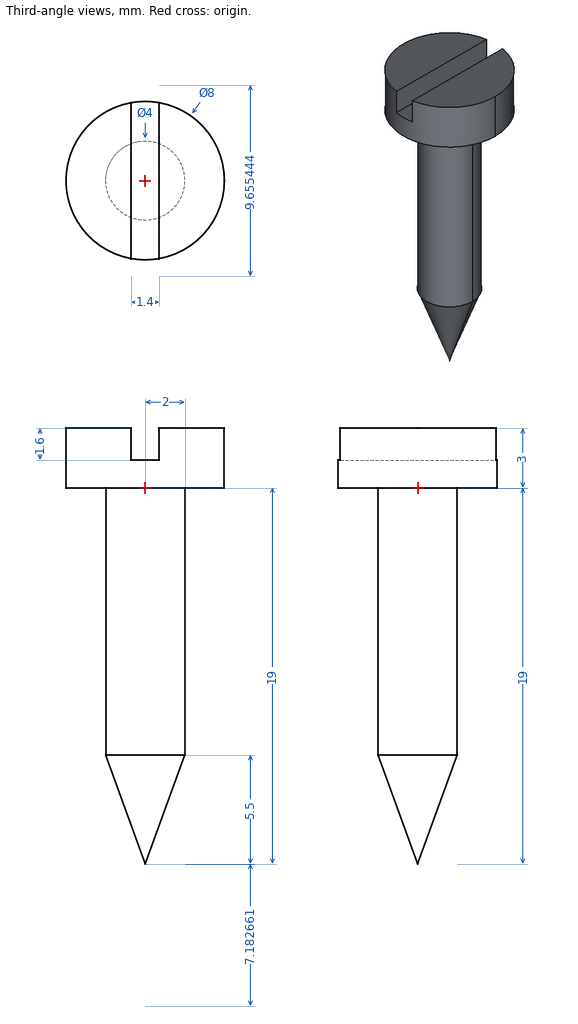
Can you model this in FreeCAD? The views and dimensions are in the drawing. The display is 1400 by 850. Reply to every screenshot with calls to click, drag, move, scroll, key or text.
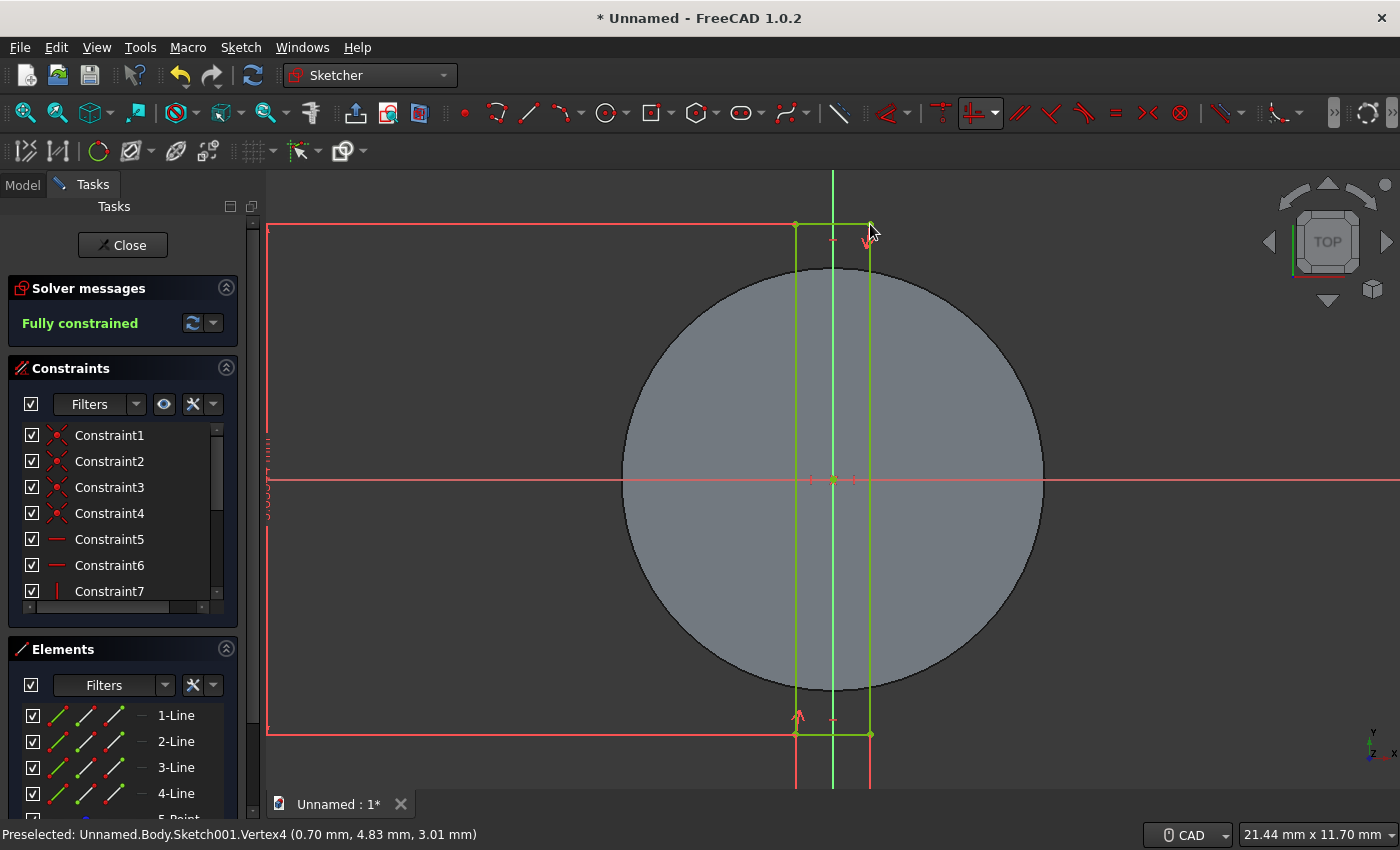
click(123, 245)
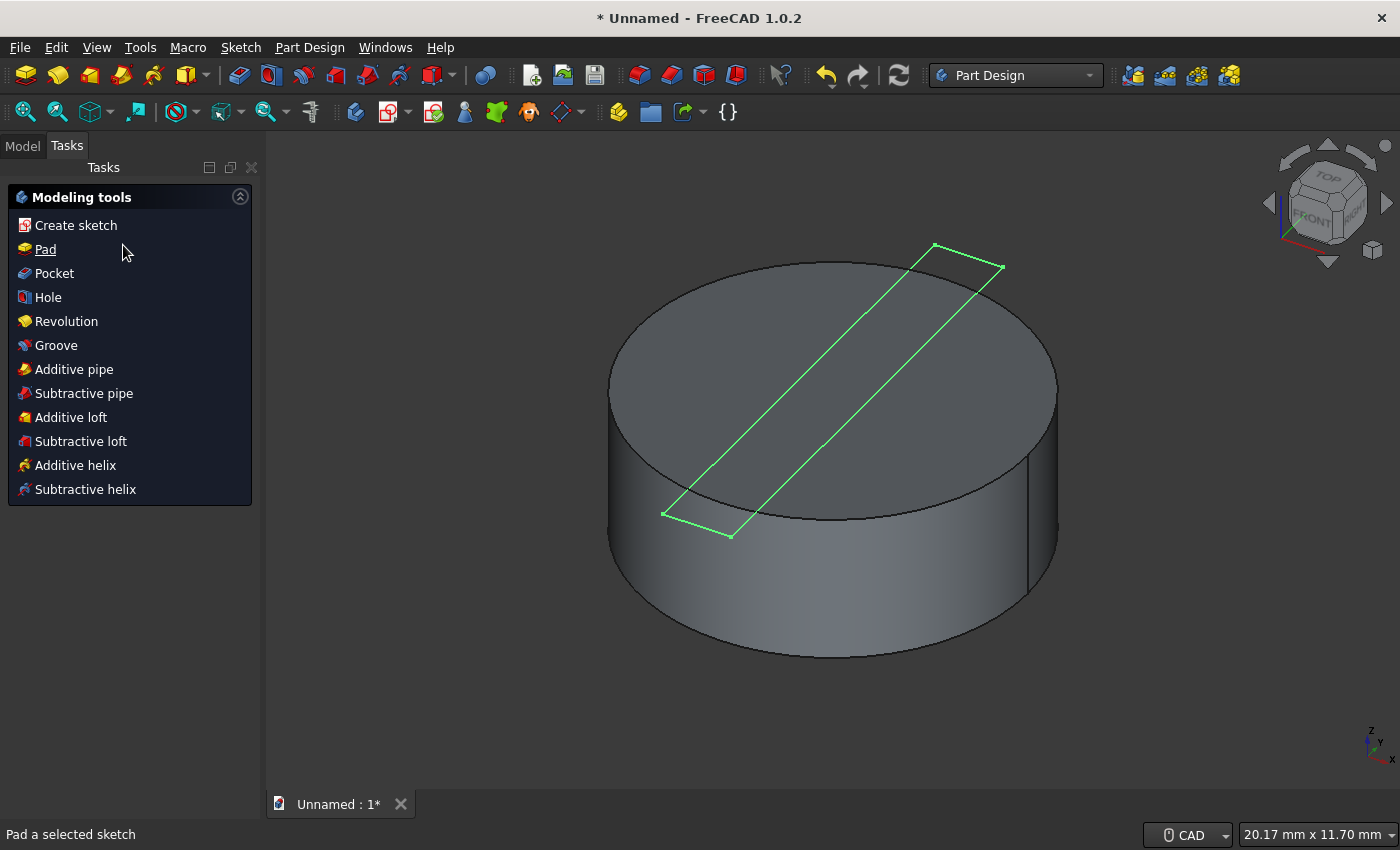
click(240, 76)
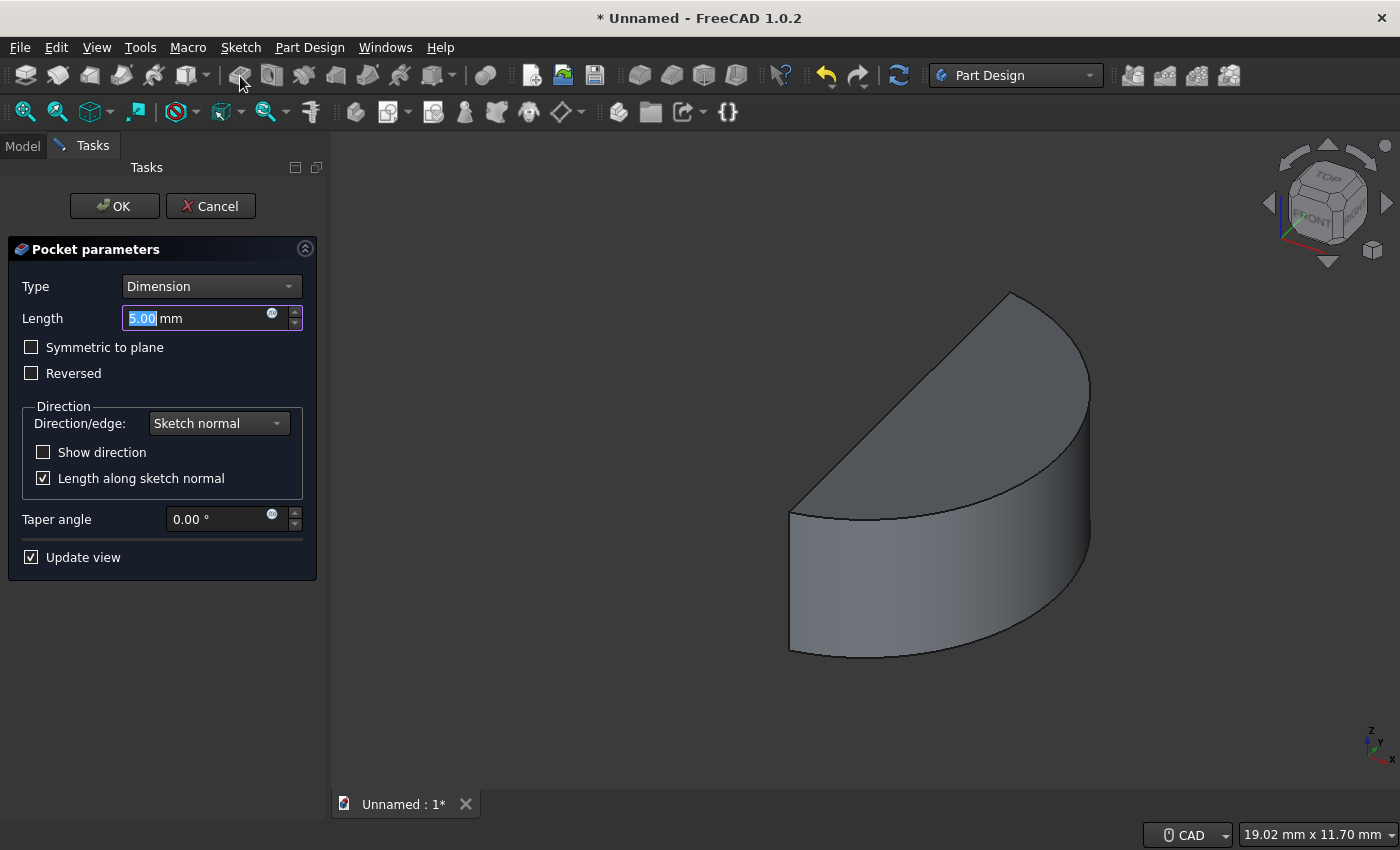
text(1.6)
key(Tab)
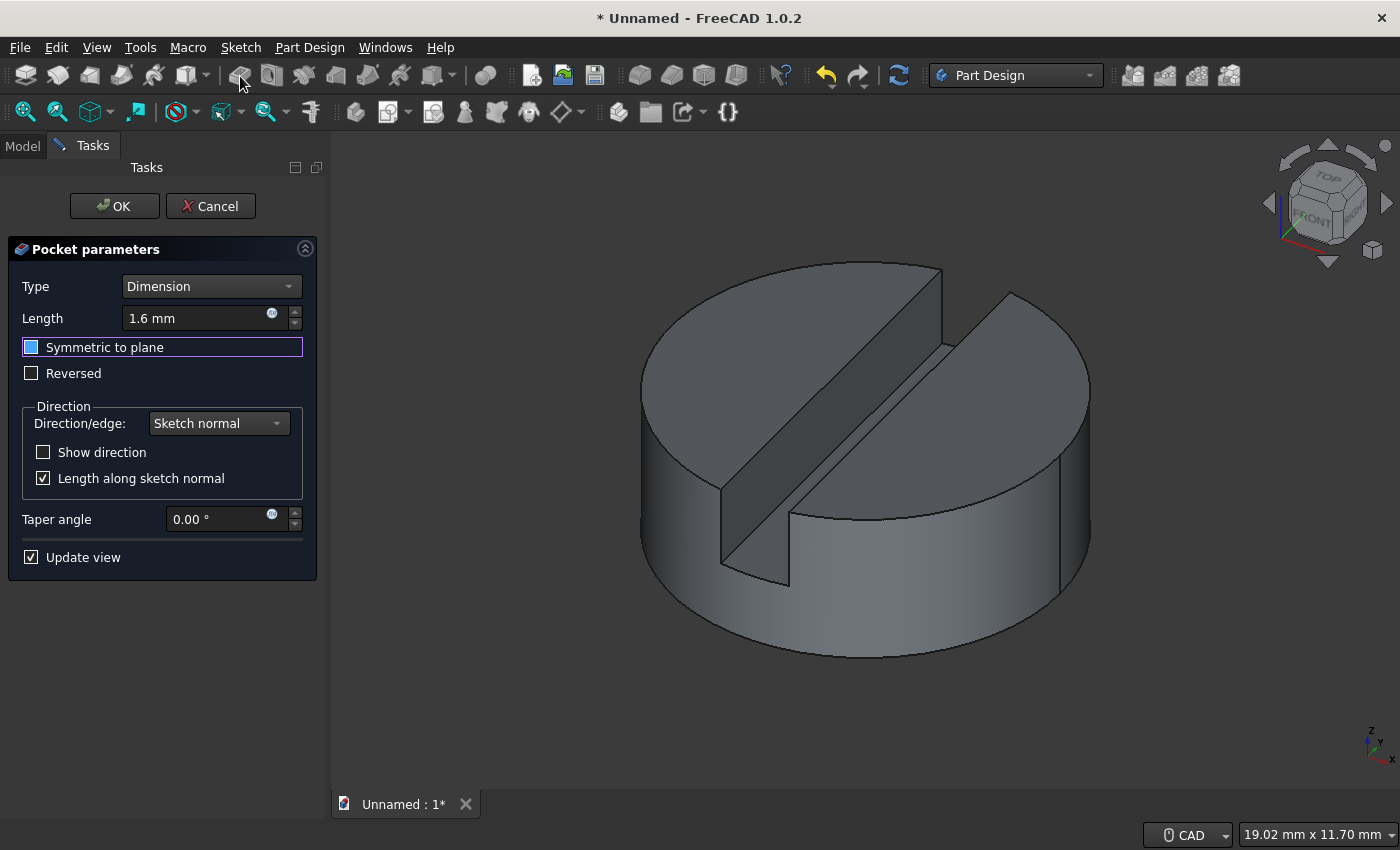
click(115, 206)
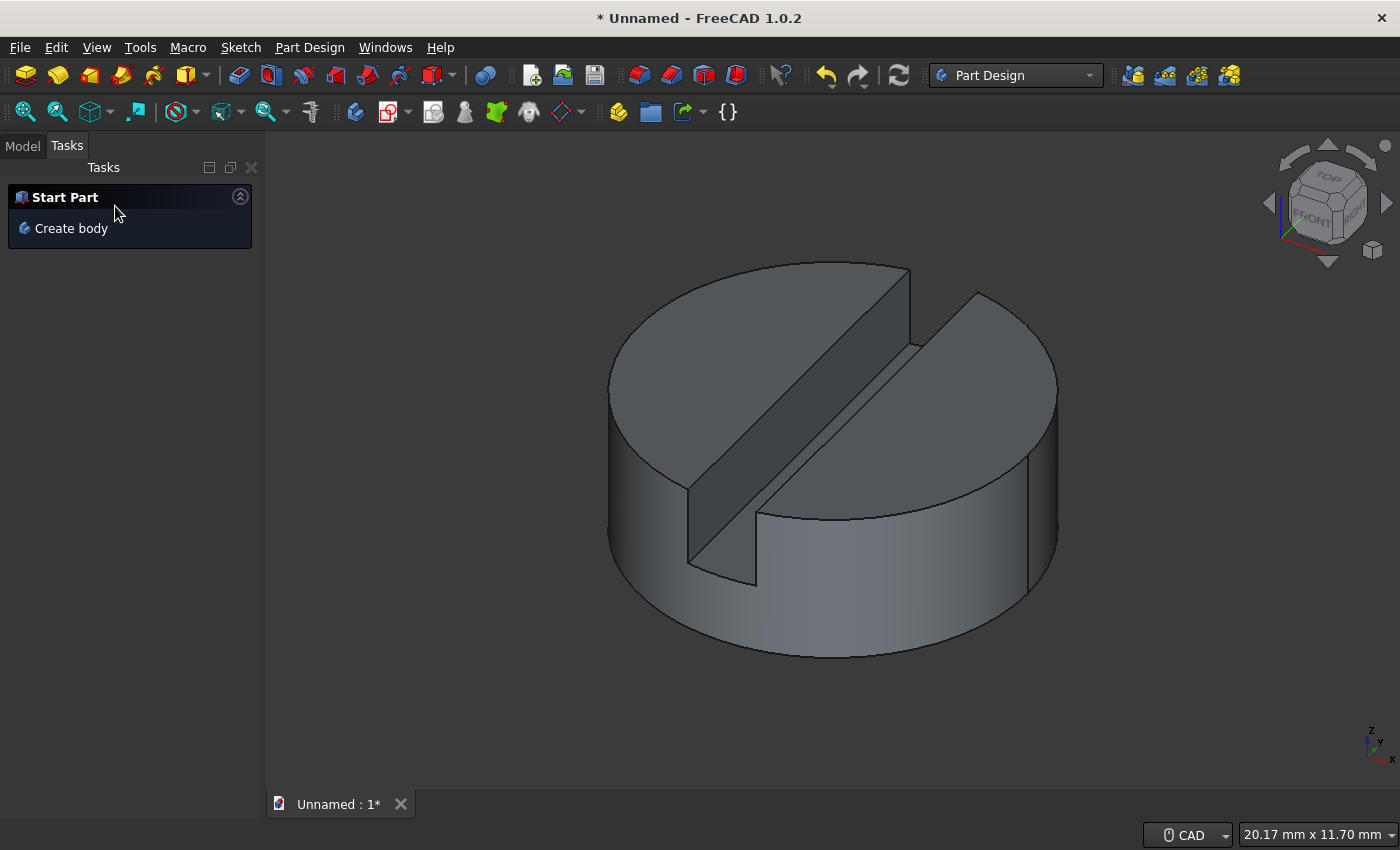
click(388, 112)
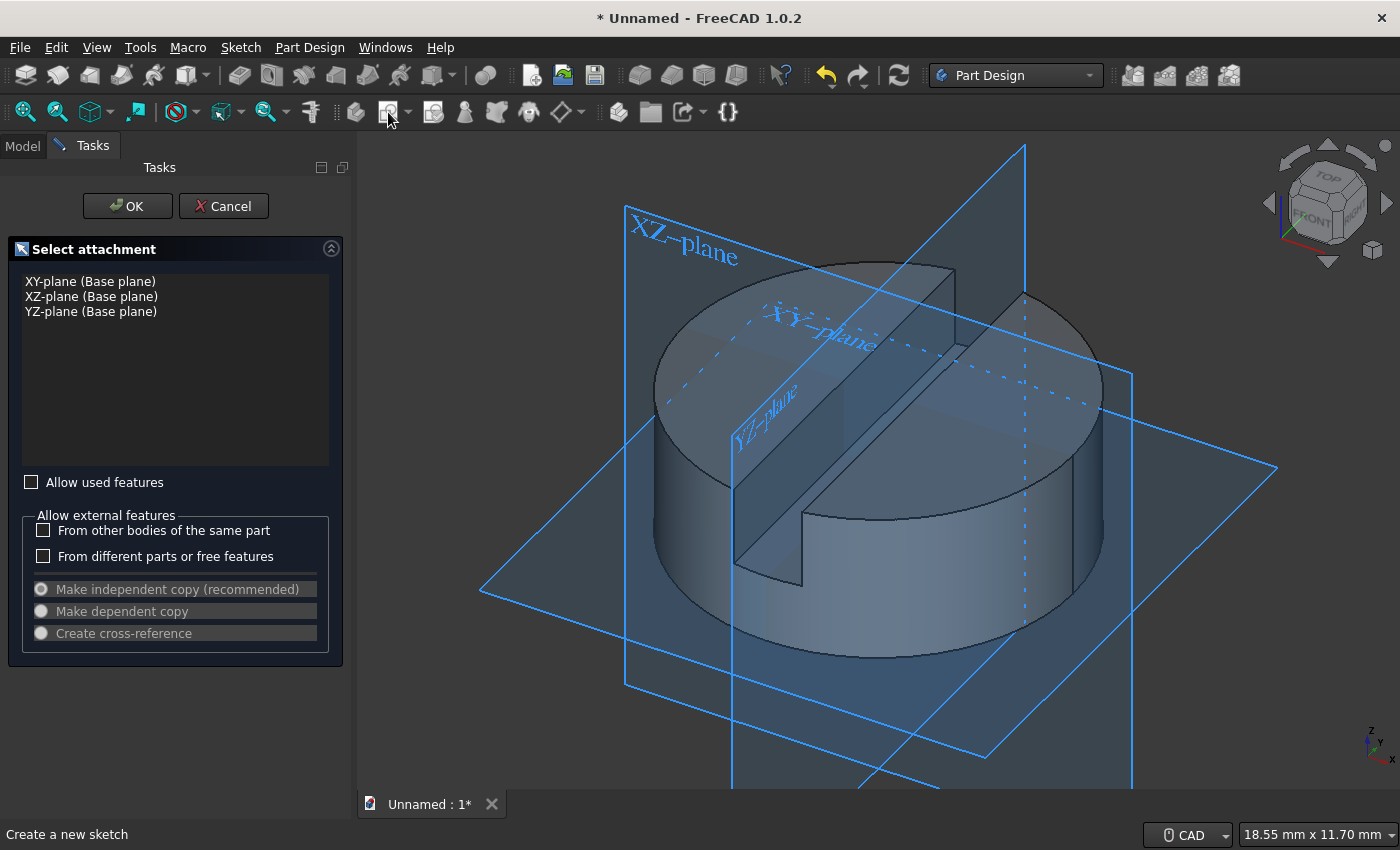
click(82, 282)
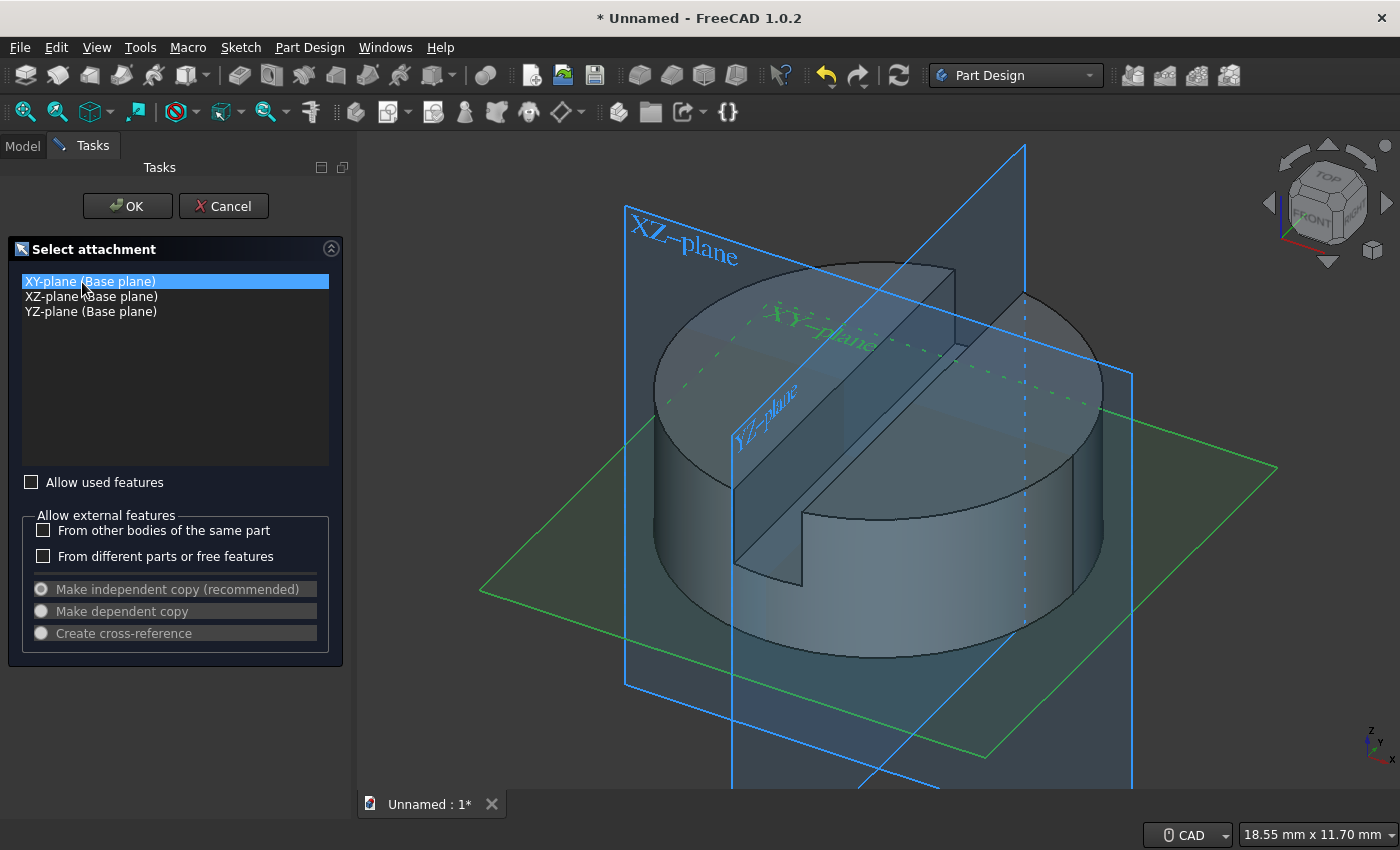
click(128, 206)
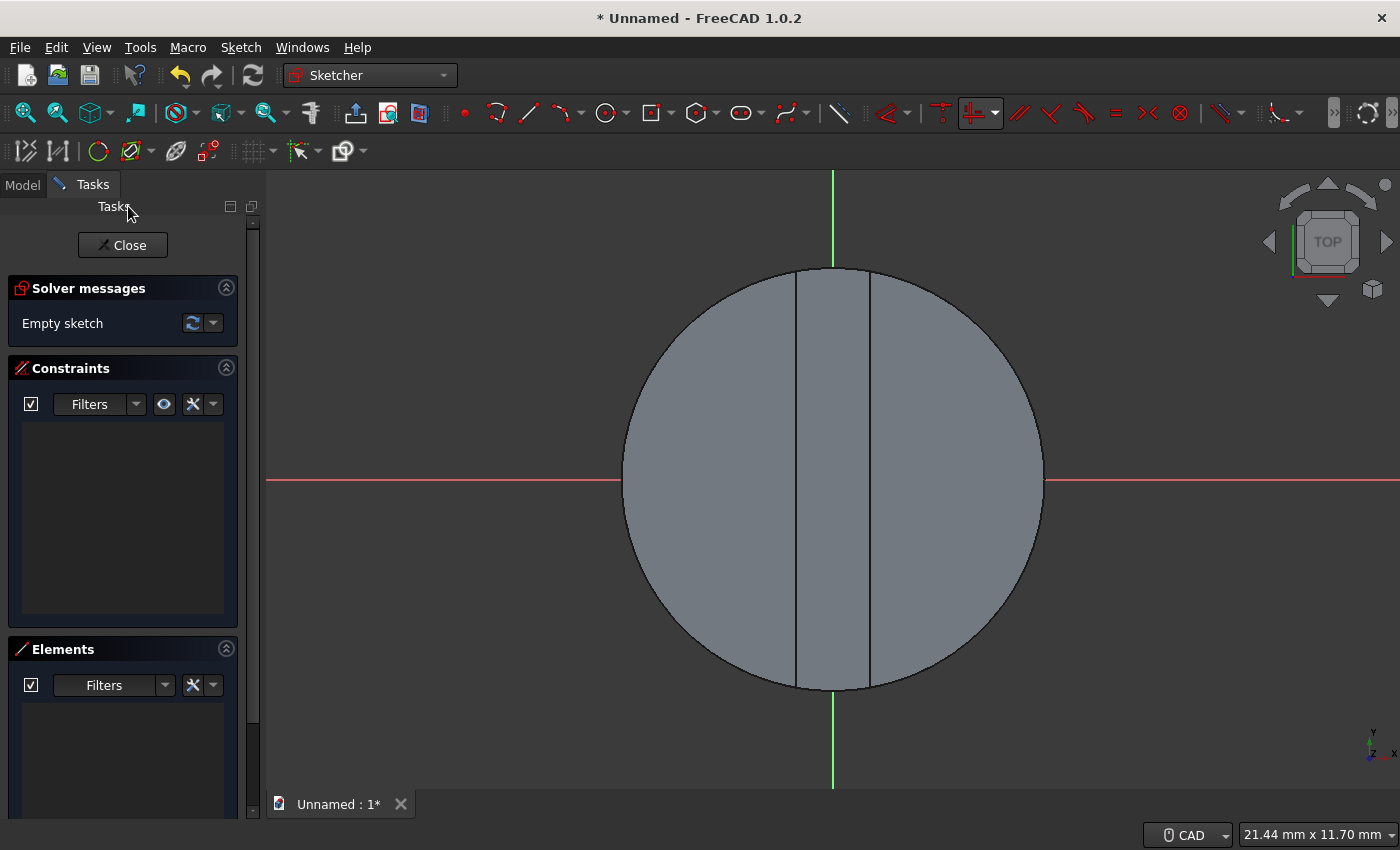
key(q)
key(s)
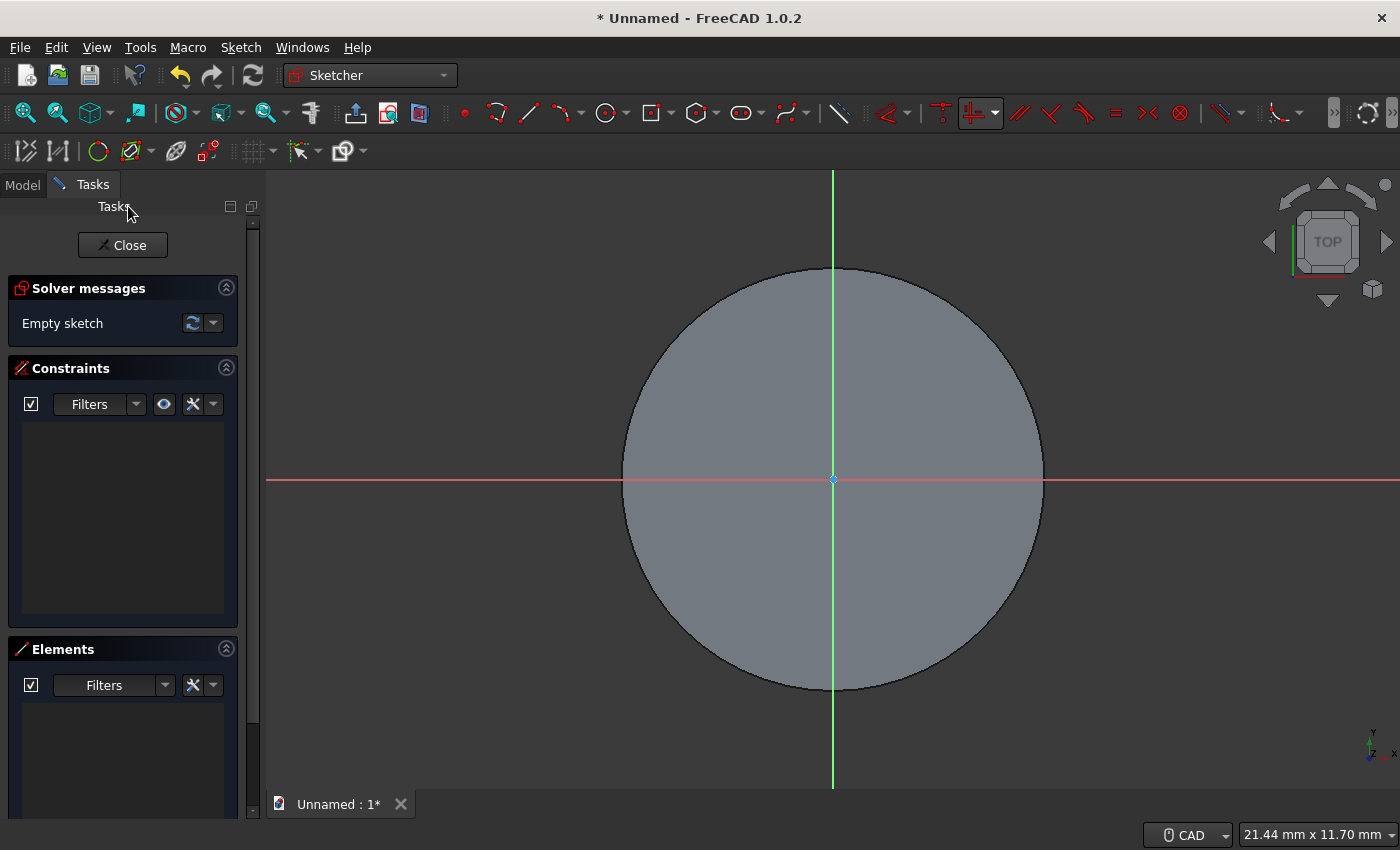
scroll(916, 480, up, 3)